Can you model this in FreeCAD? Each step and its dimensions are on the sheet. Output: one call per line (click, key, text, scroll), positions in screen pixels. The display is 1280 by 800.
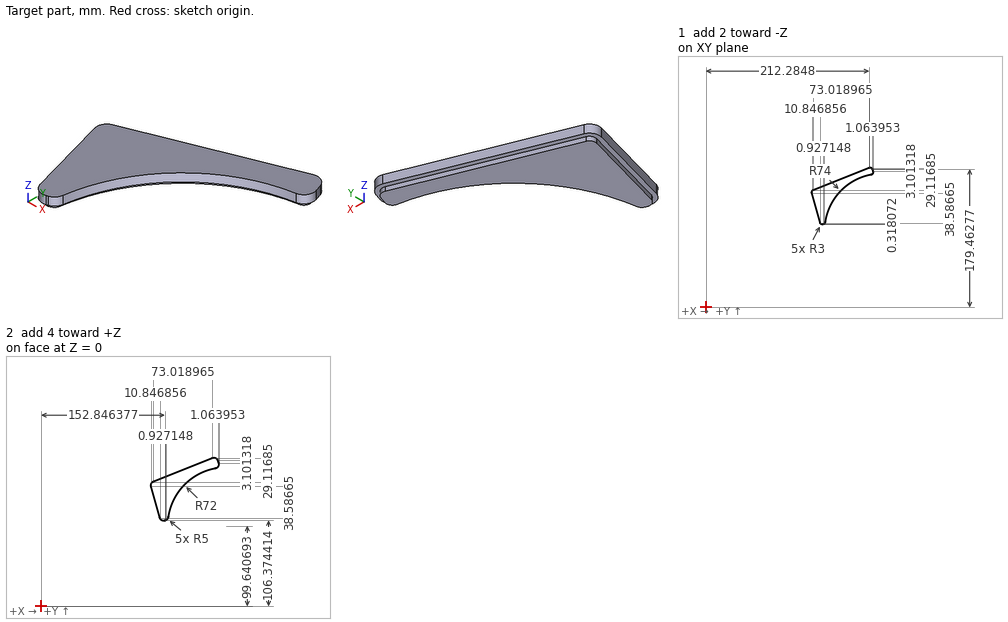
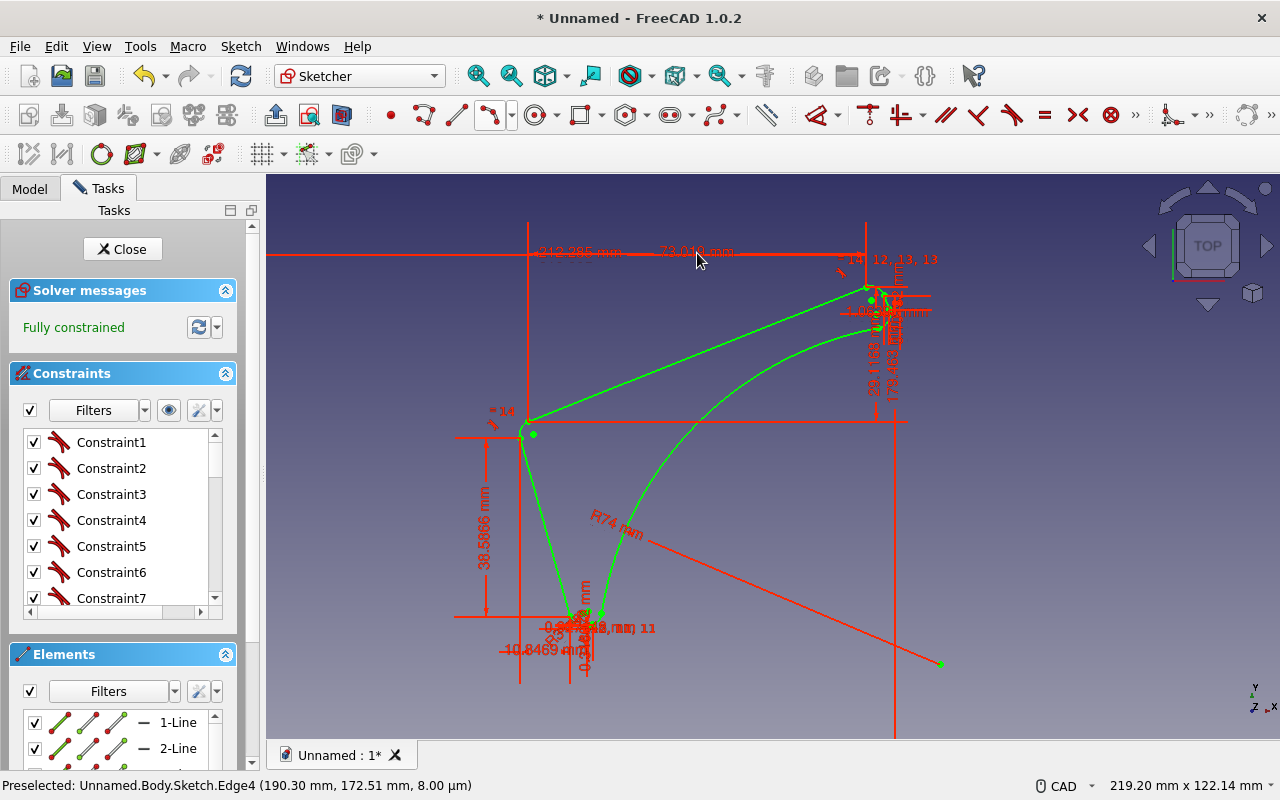
click(123, 249)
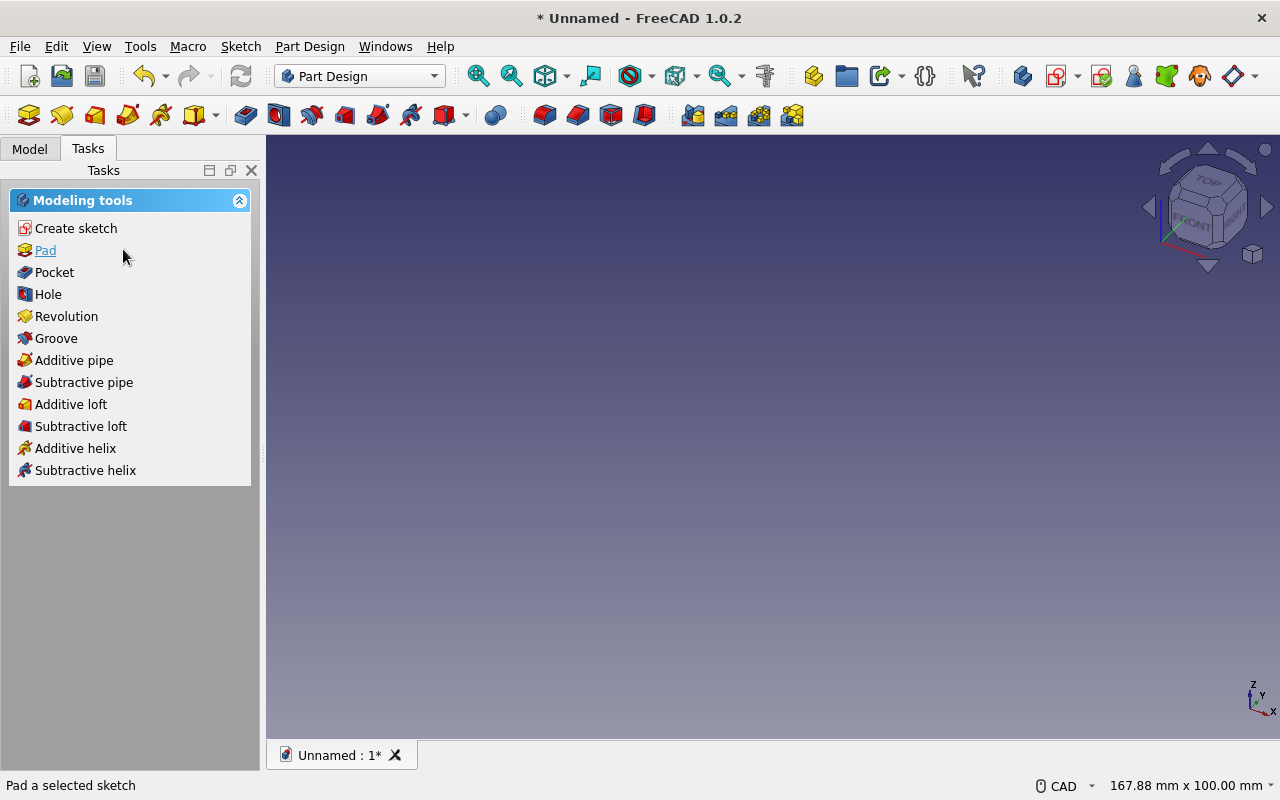
click(29, 116)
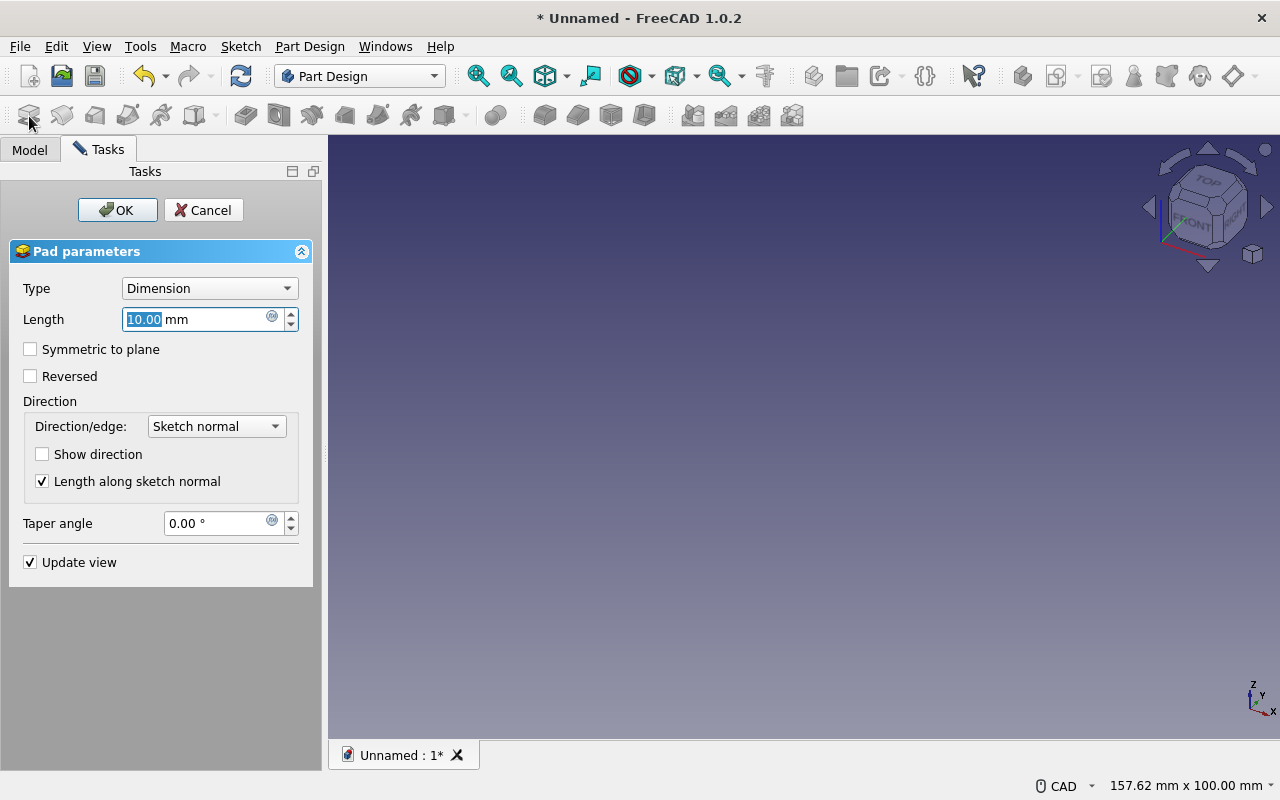
text(2)
key(Tab)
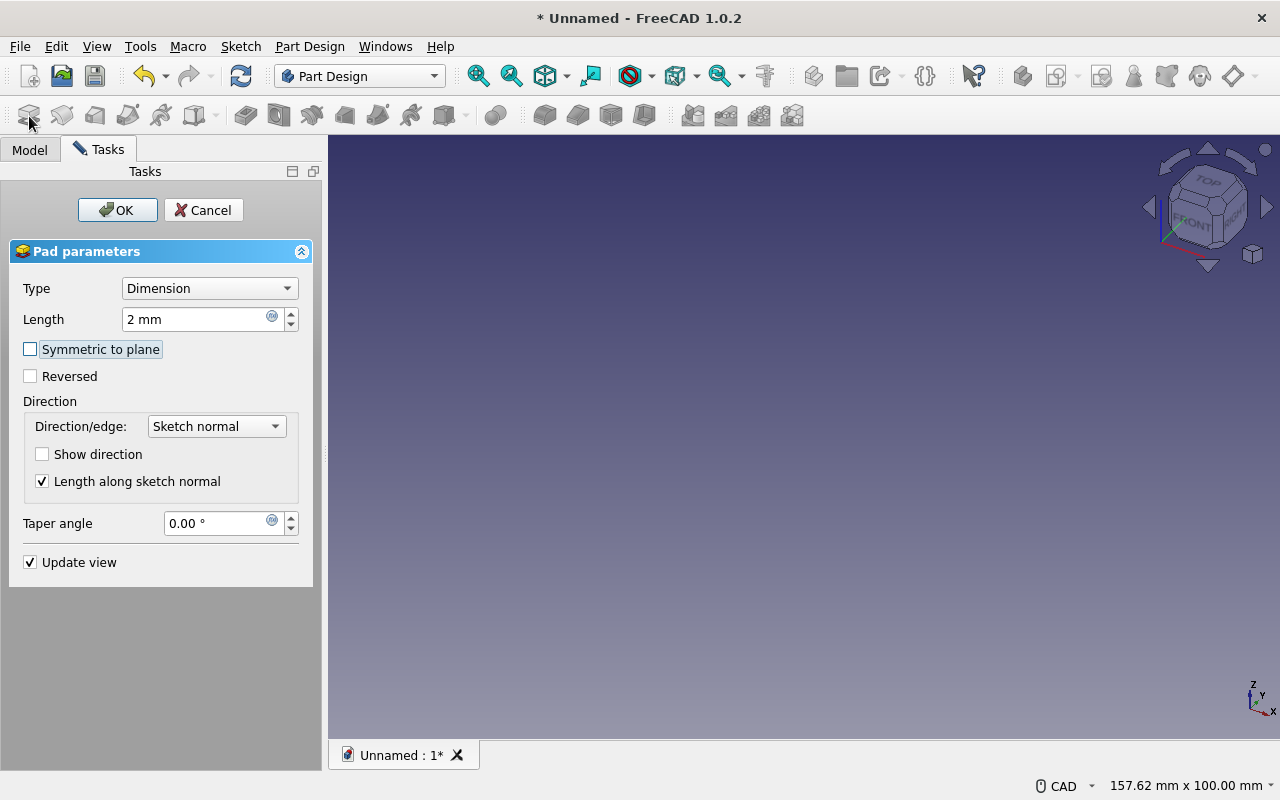
click(31, 376)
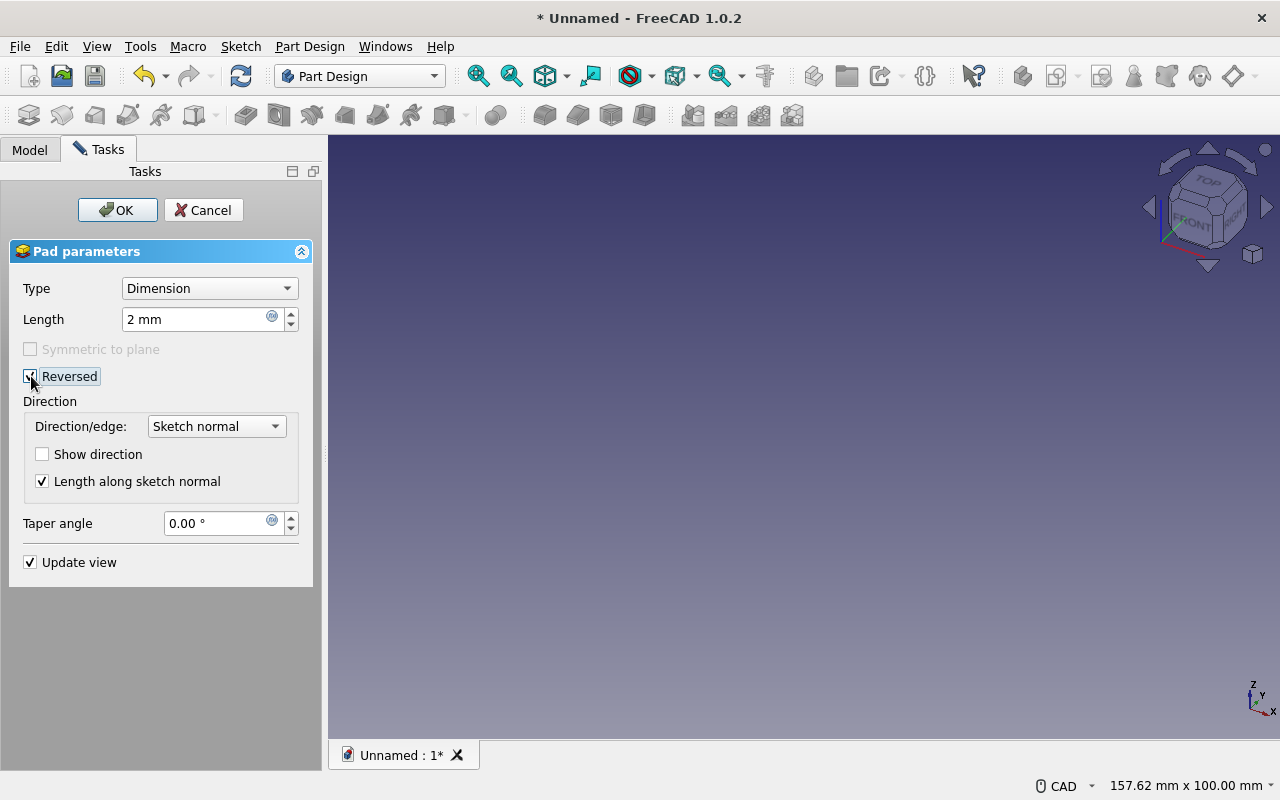
click(118, 210)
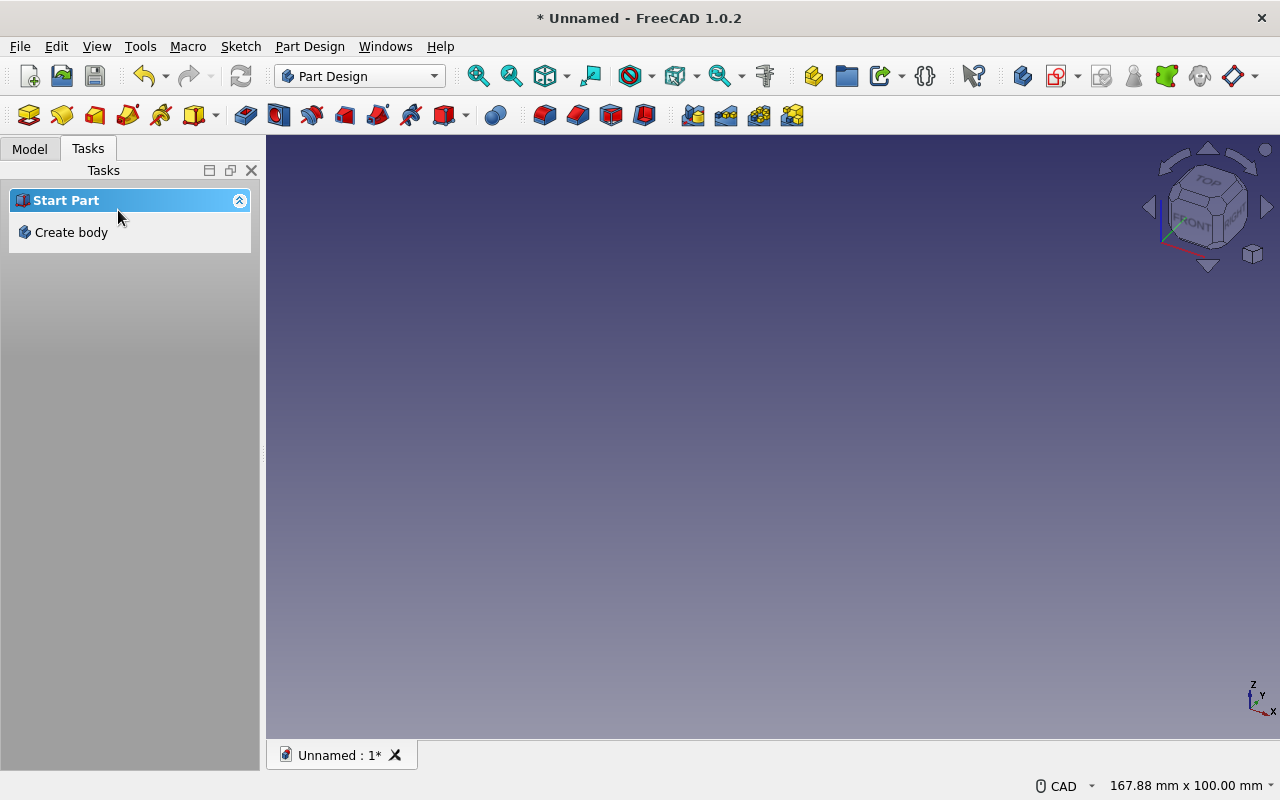
click(479, 76)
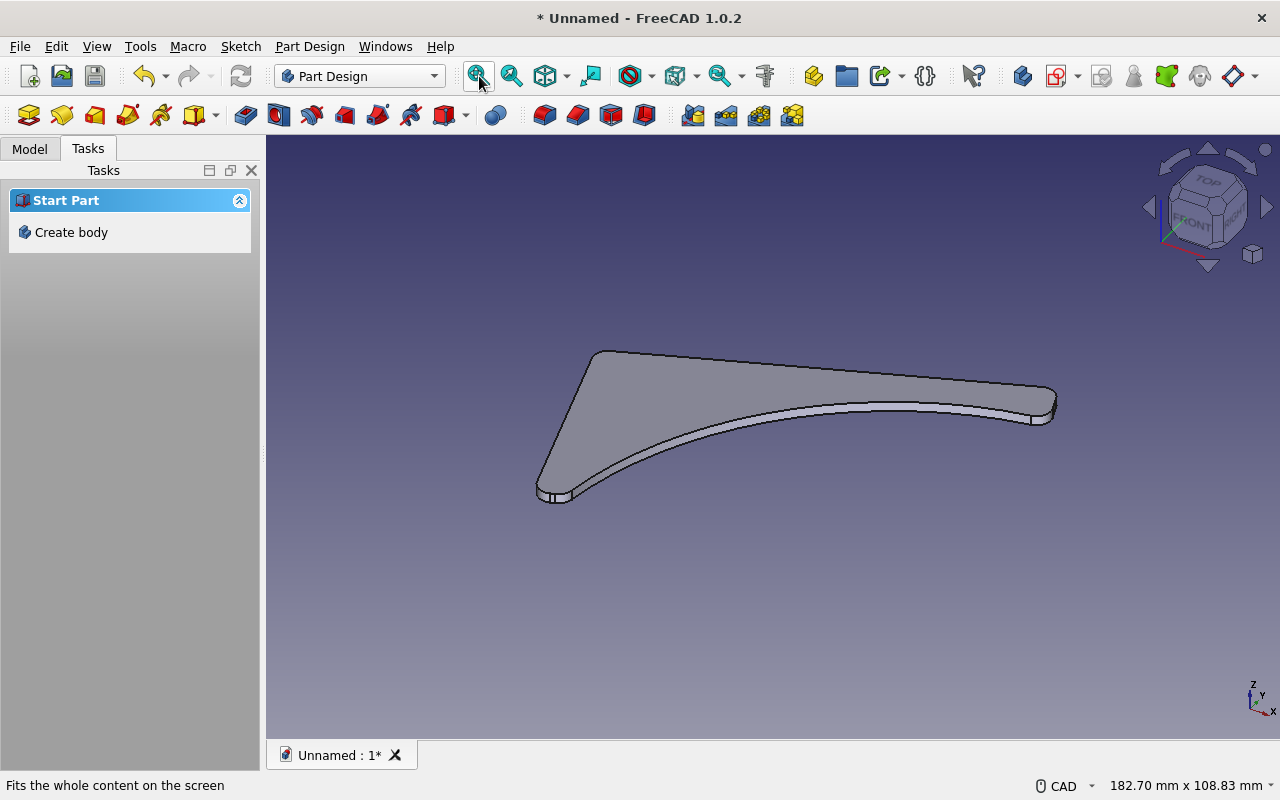
click(663, 395)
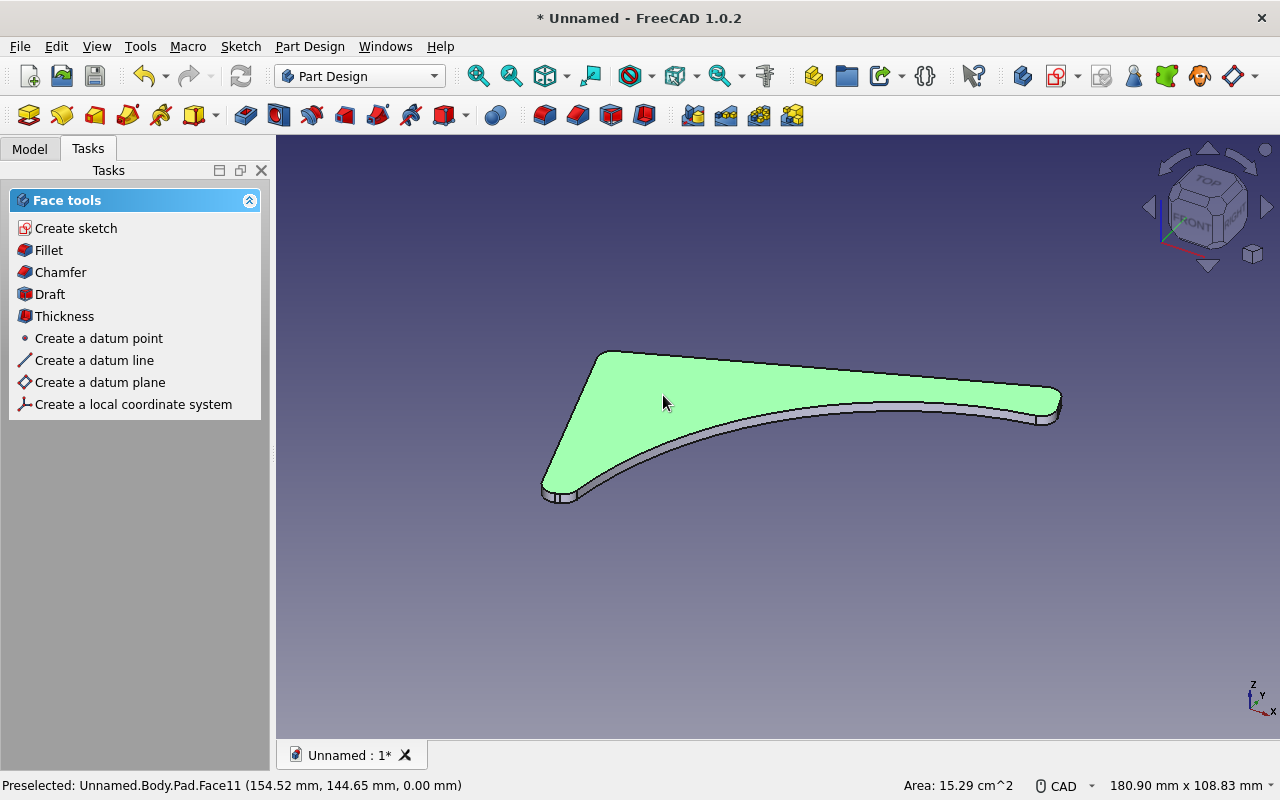
click(1056, 76)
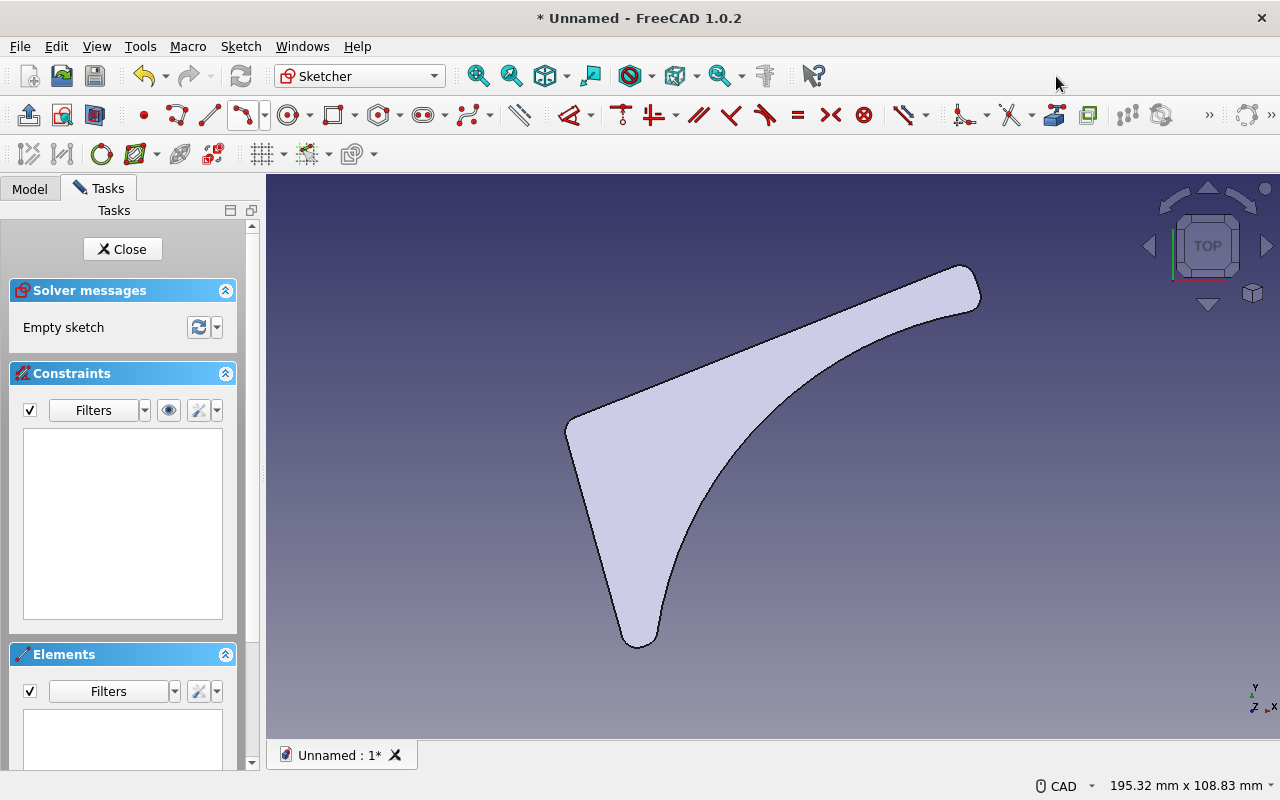
click(210, 116)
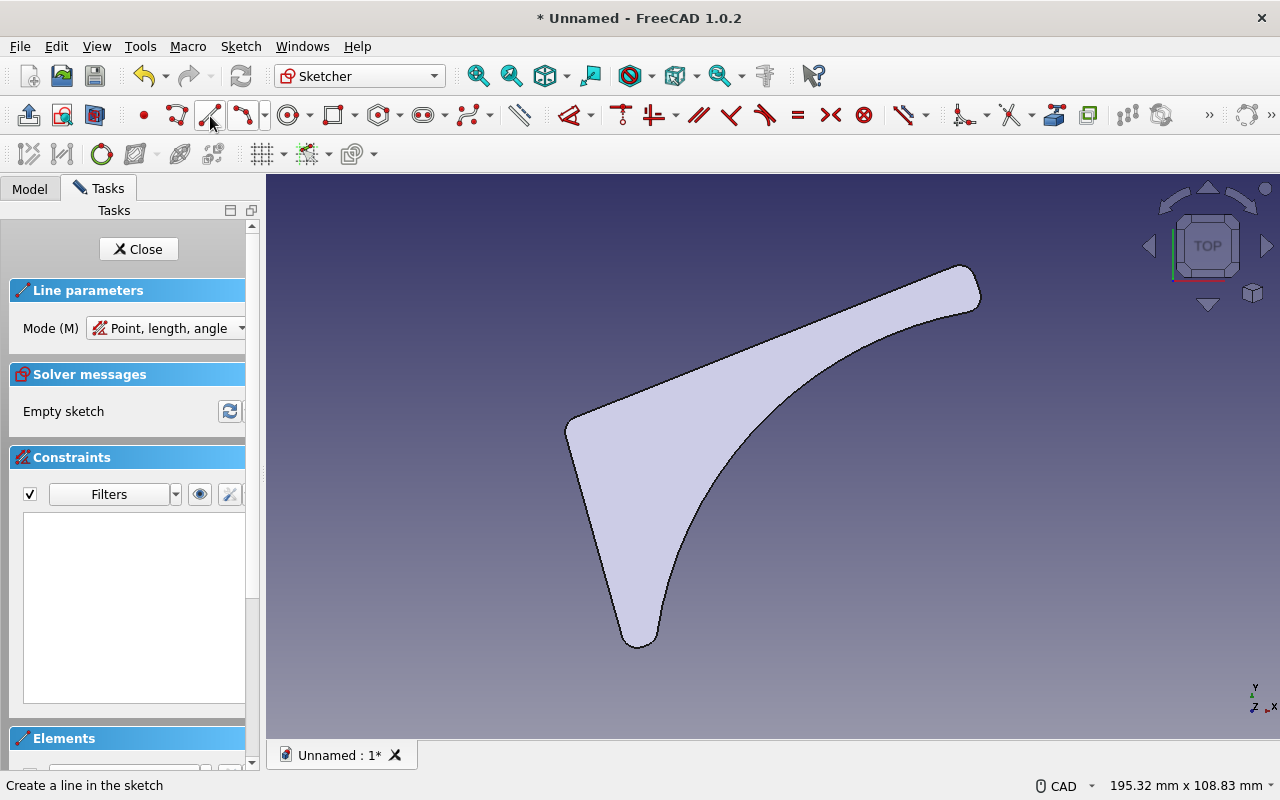
click(645, 657)